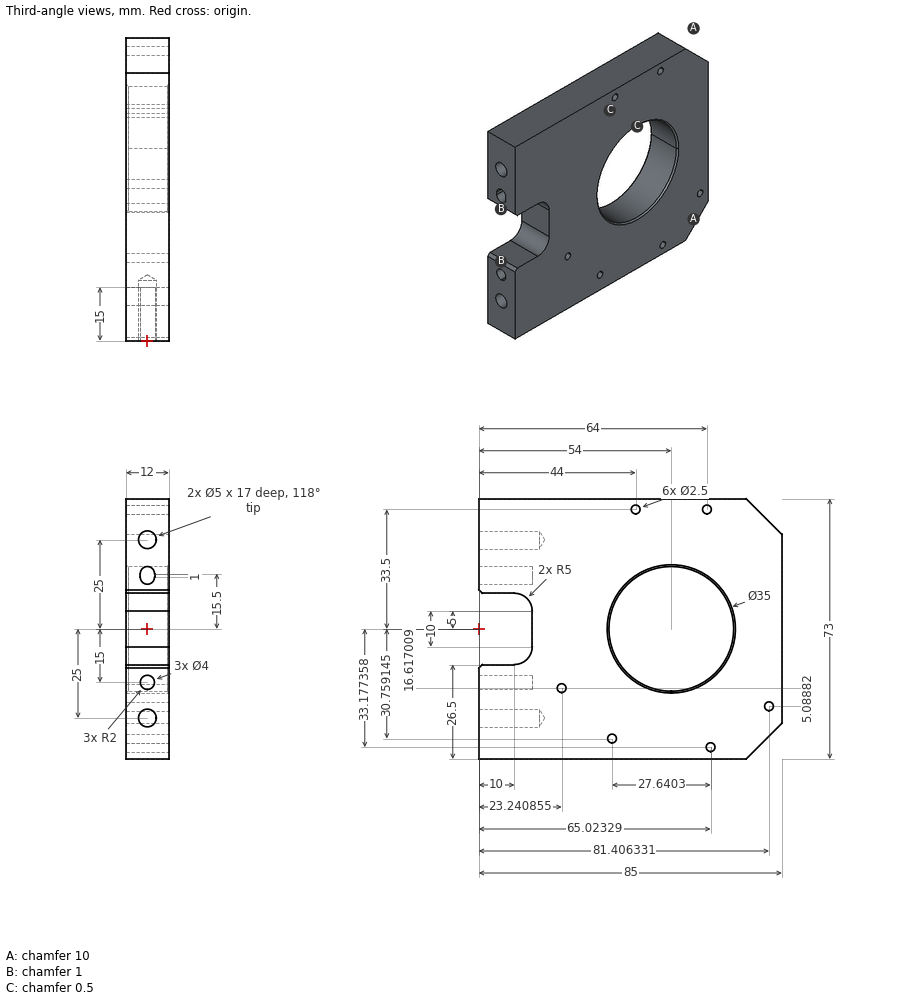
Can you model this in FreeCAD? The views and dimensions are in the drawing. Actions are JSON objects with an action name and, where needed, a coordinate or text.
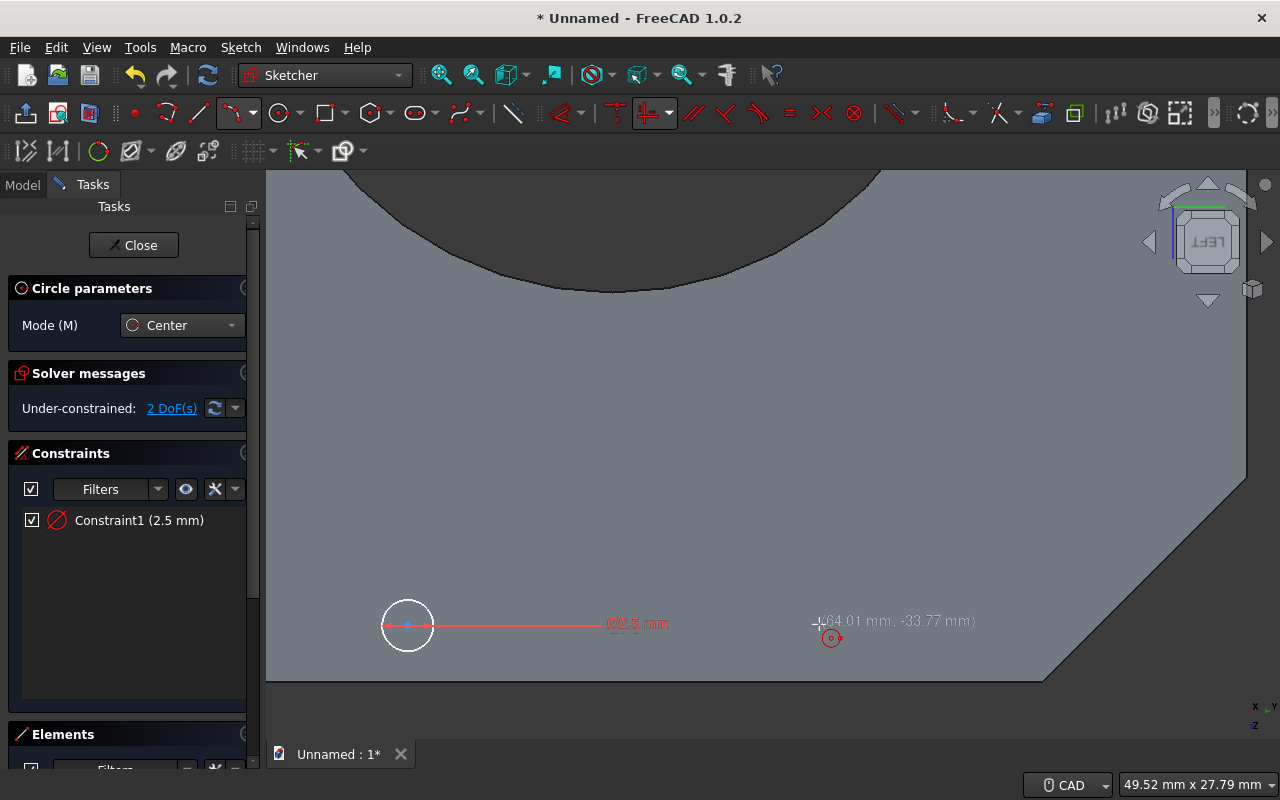
{"action": "scroll", "coordinate": [820, 624], "scroll_direction": "down", "scroll_amount": 7}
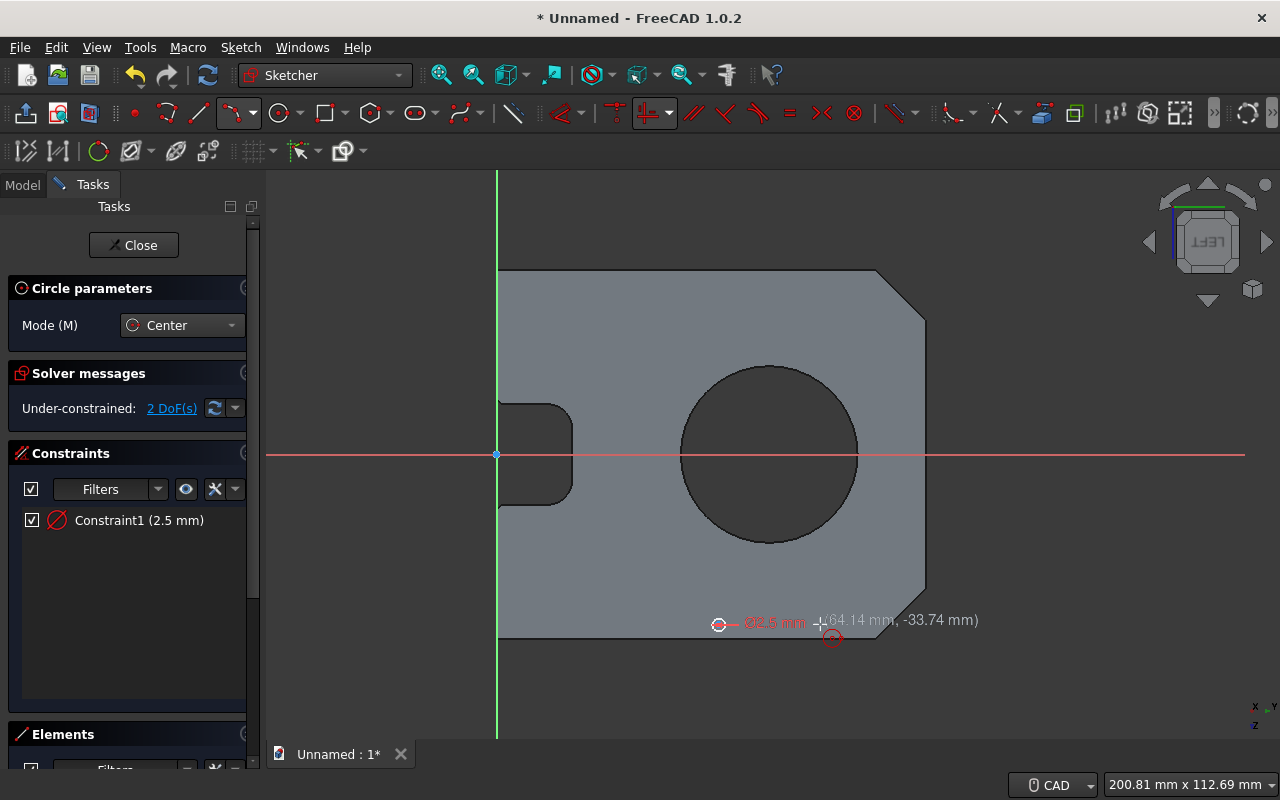
{"action": "left_click", "coordinate": [820, 624]}
{"action": "mouse_move", "coordinate": [824, 619]}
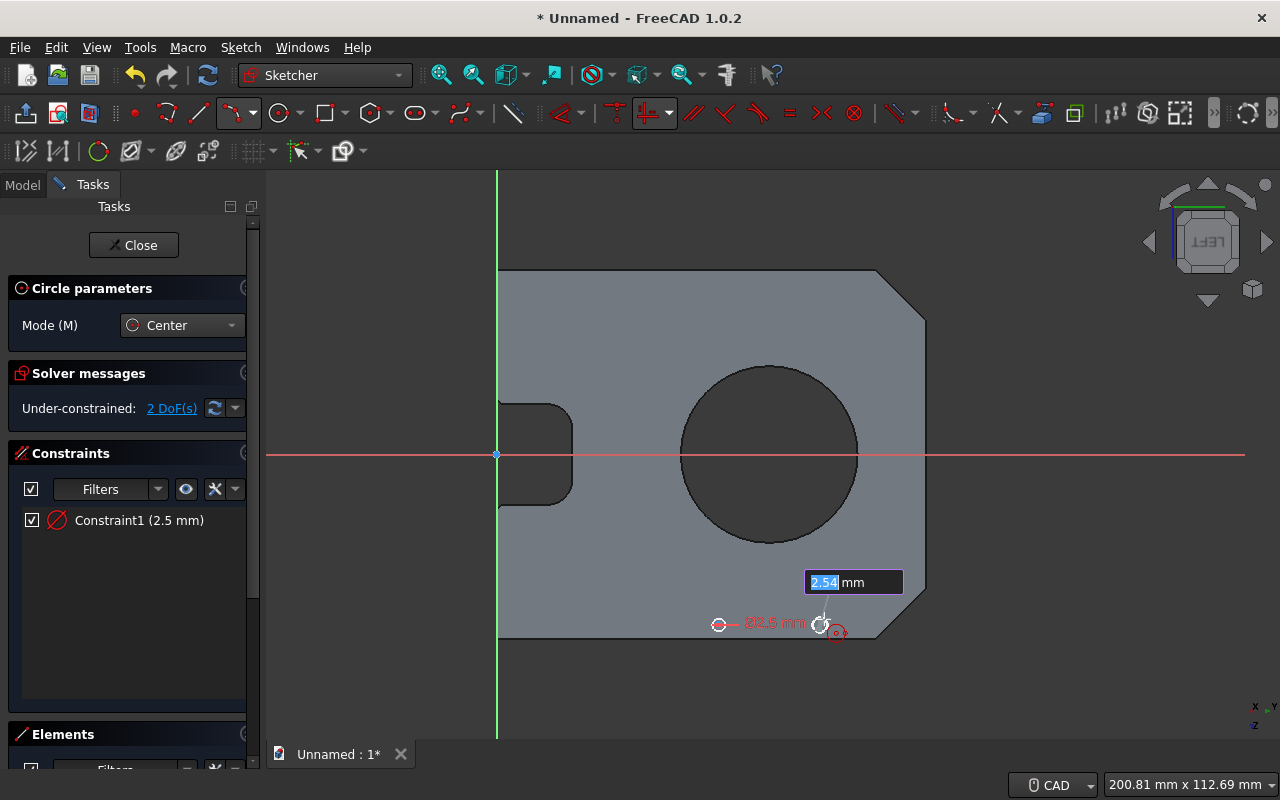
{"action": "type", "text": "2.5"}
{"action": "key", "text": "Return"}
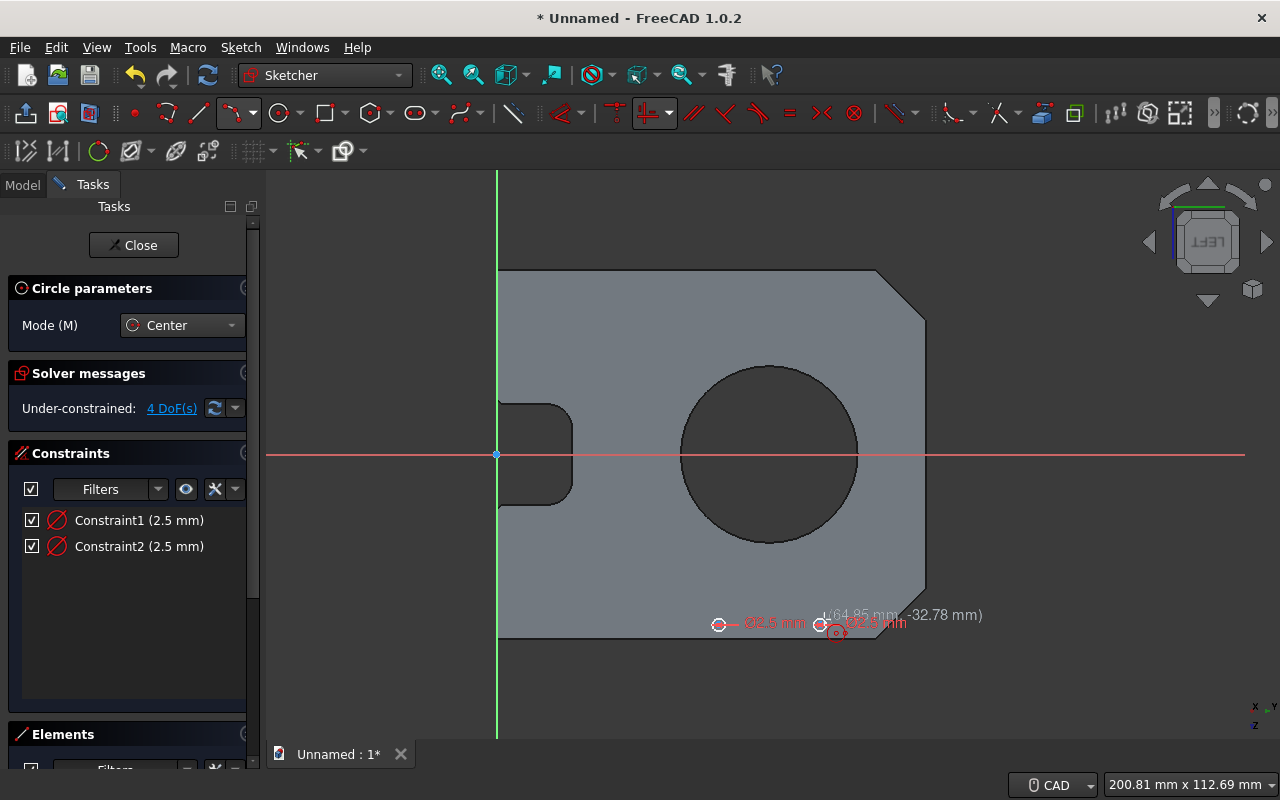
{"action": "scroll", "coordinate": [614, 371], "scroll_direction": "up", "scroll_amount": 7}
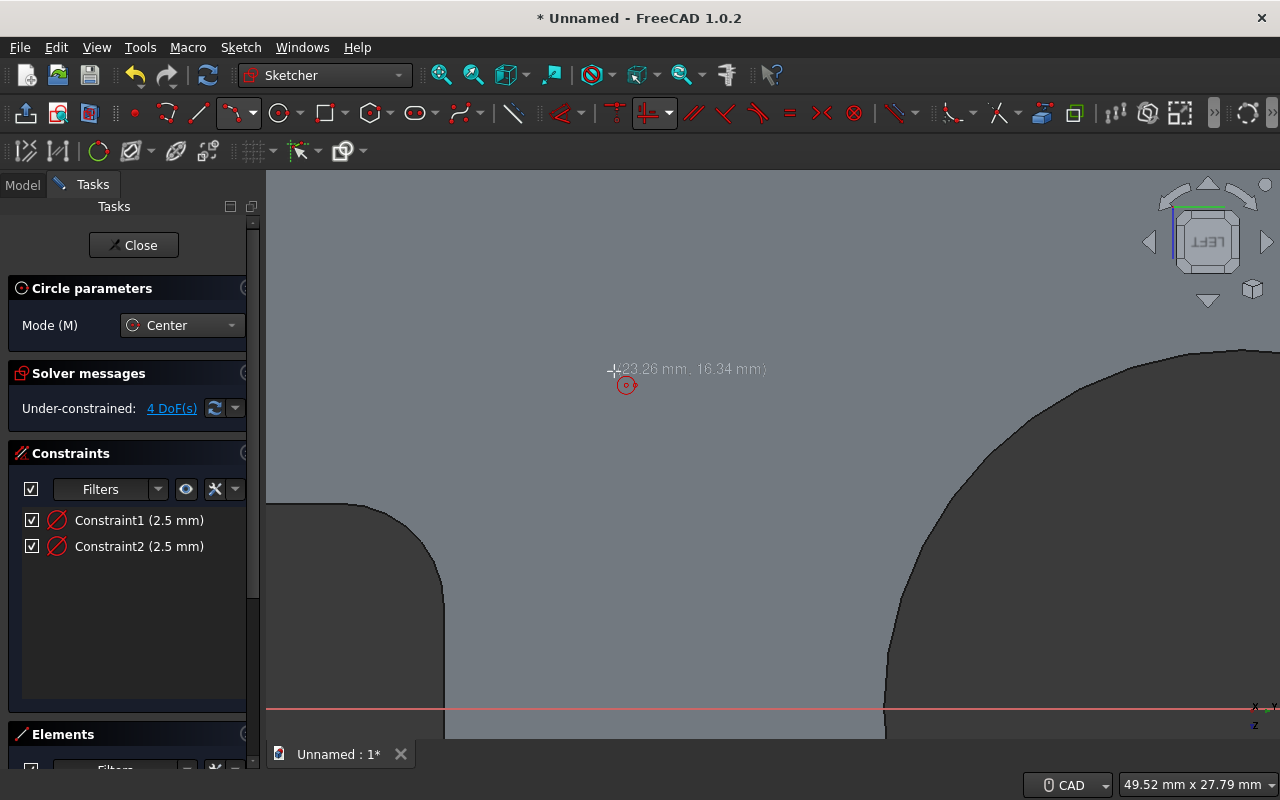
{"action": "scroll", "coordinate": [613, 370], "scroll_direction": "down", "scroll_amount": 7}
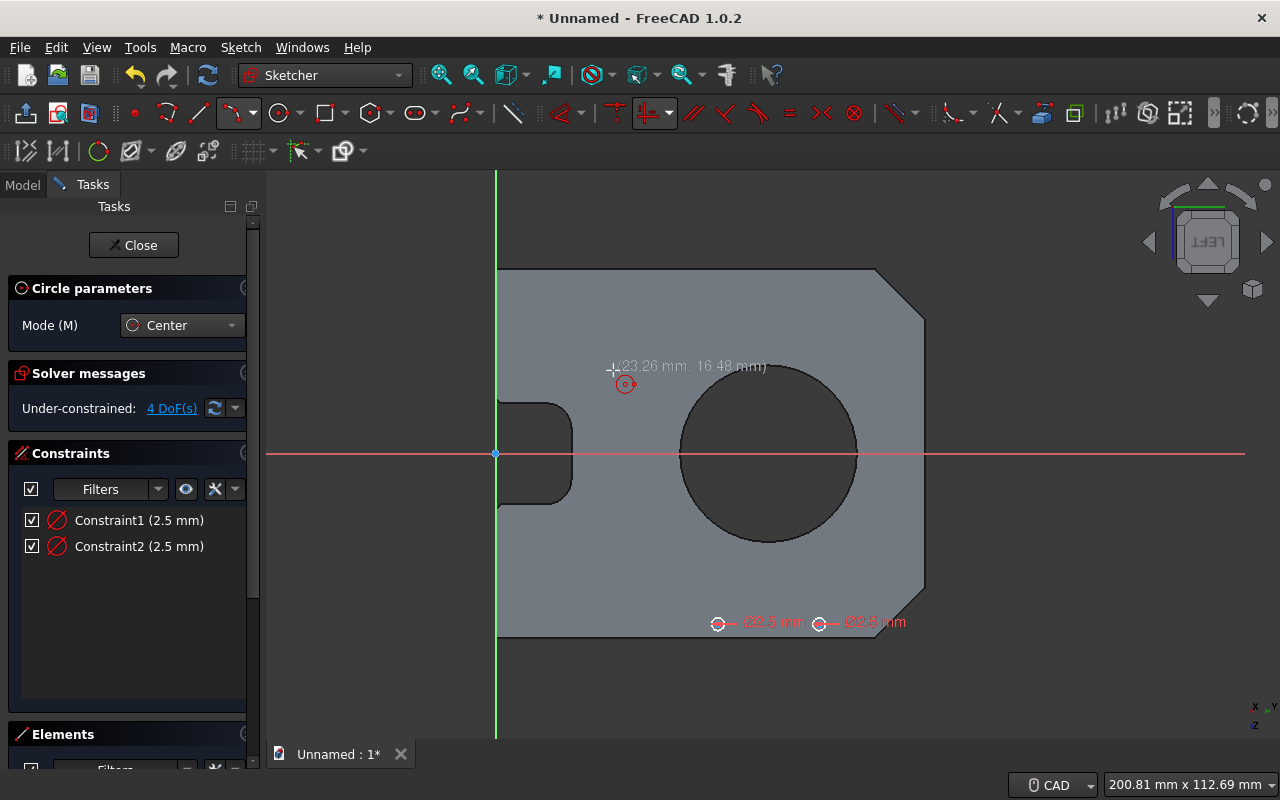
{"action": "left_click", "coordinate": [613, 370]}
{"action": "mouse_move", "coordinate": [618, 365]}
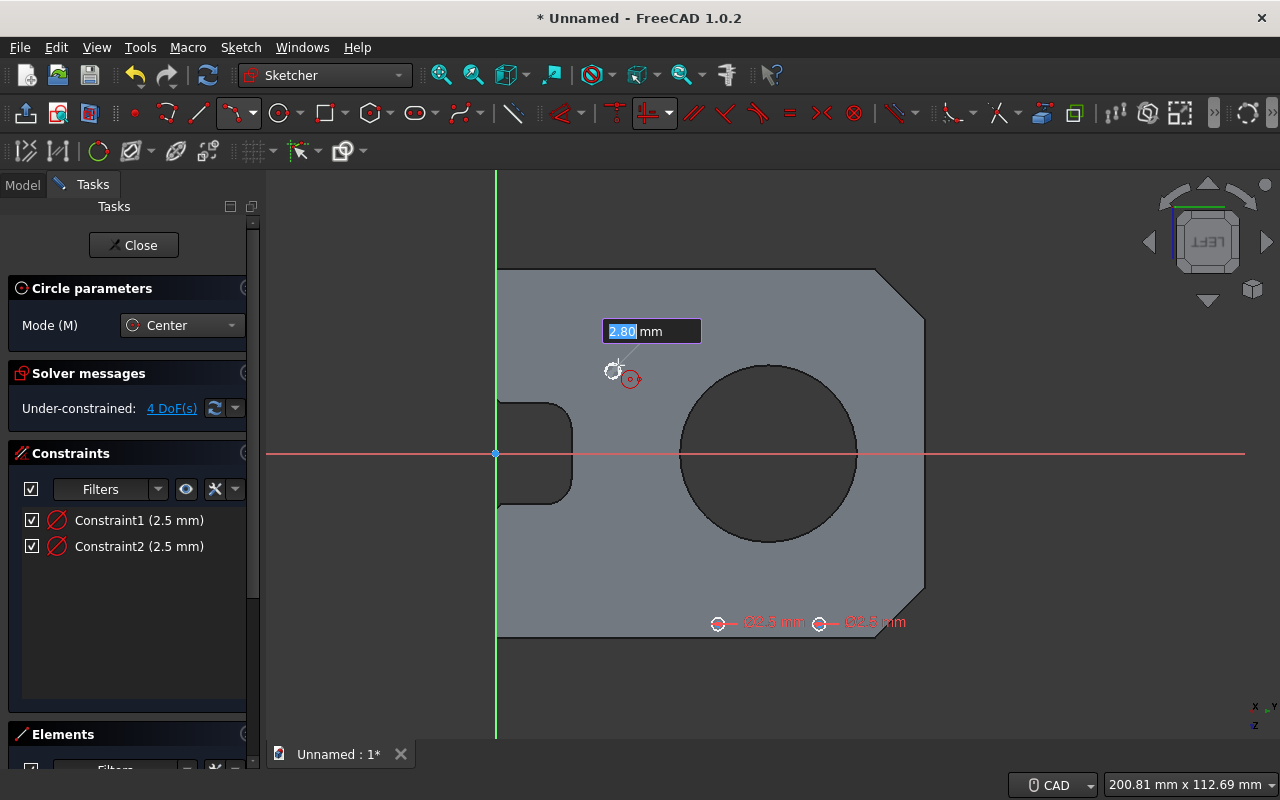
{"action": "type", "text": "2.5"}
{"action": "key", "text": "Return"}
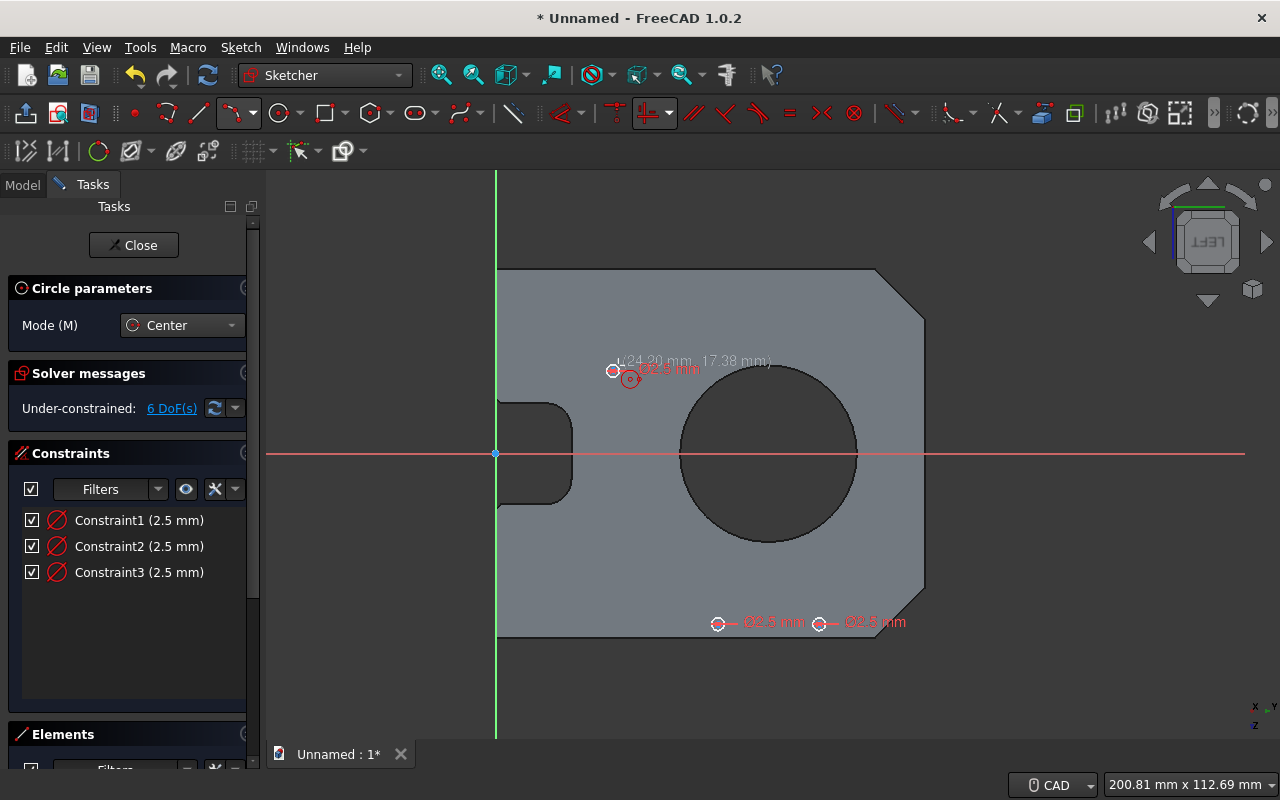
{"action": "scroll", "coordinate": [685, 298], "scroll_direction": "up", "scroll_amount": 7}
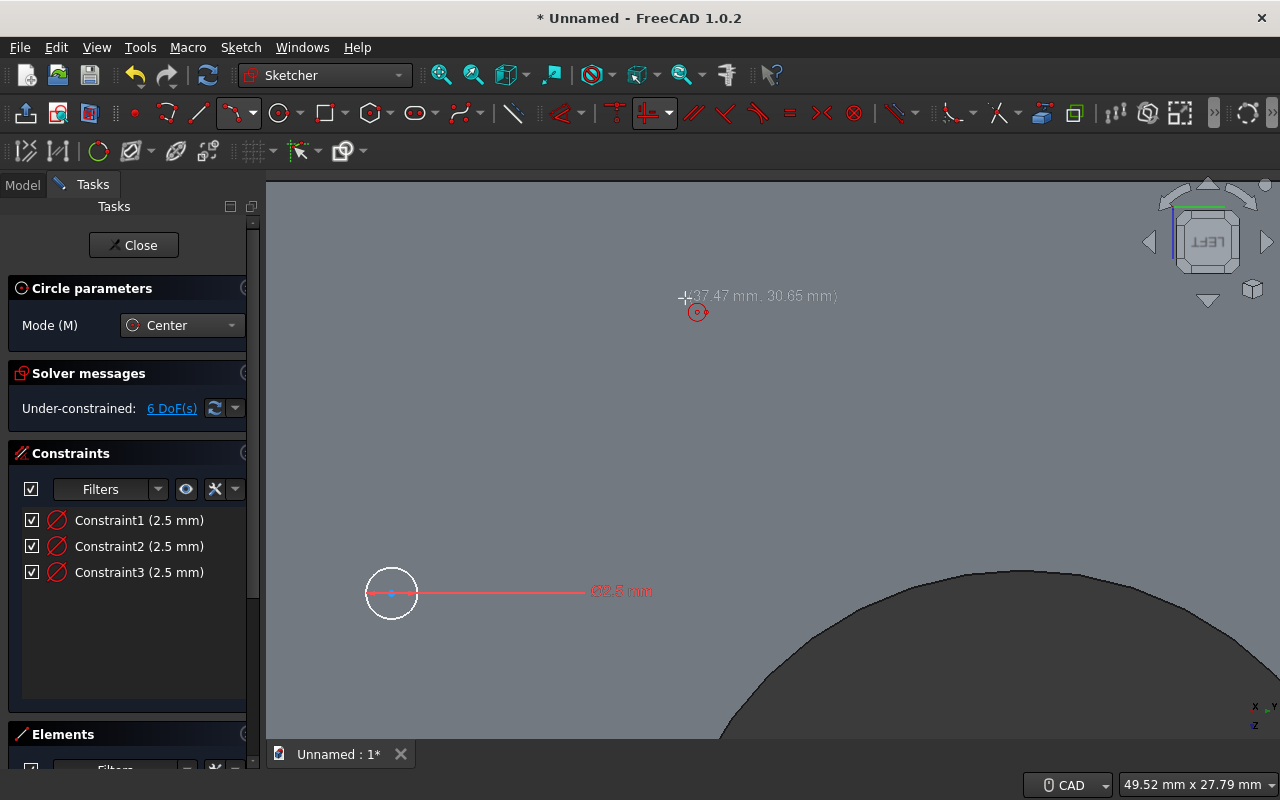
{"action": "scroll", "coordinate": [685, 298], "scroll_direction": "down", "scroll_amount": 7}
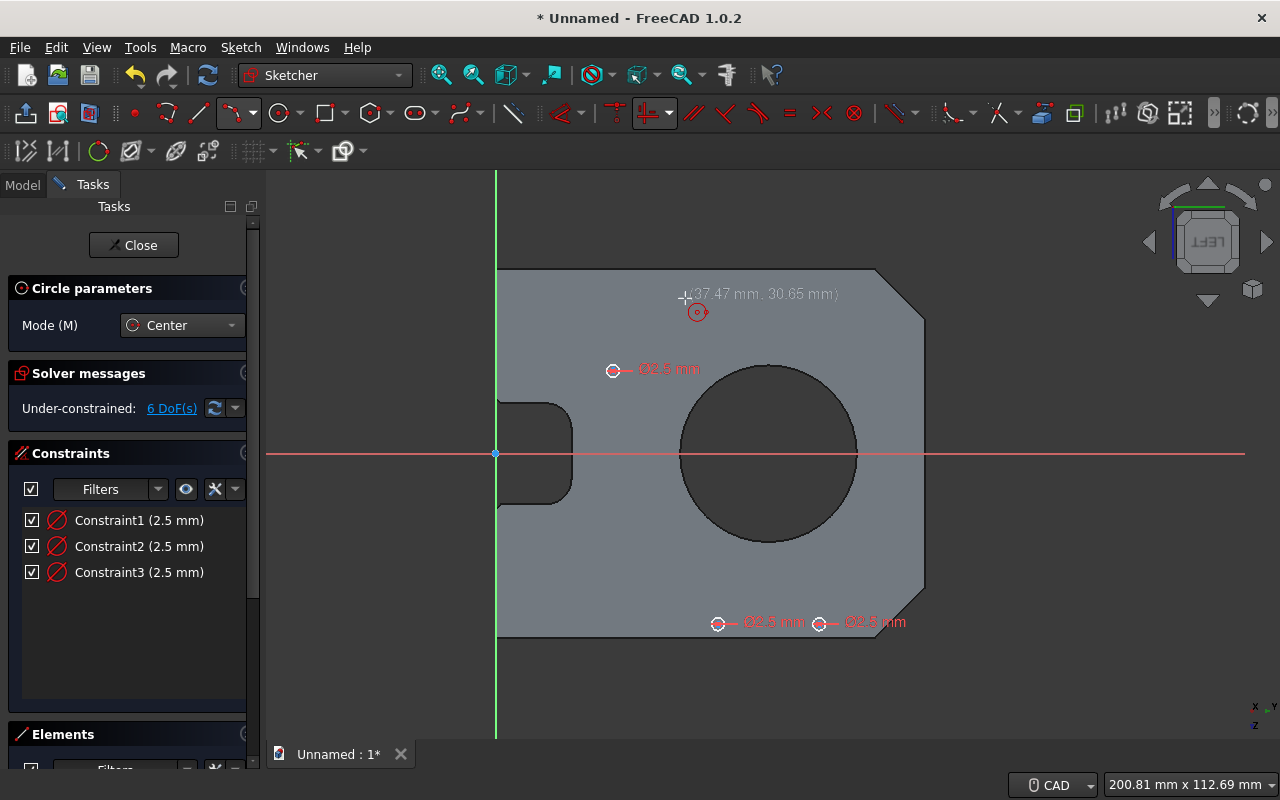
{"action": "left_click", "coordinate": [685, 298]}
{"action": "mouse_move", "coordinate": [689, 294]}